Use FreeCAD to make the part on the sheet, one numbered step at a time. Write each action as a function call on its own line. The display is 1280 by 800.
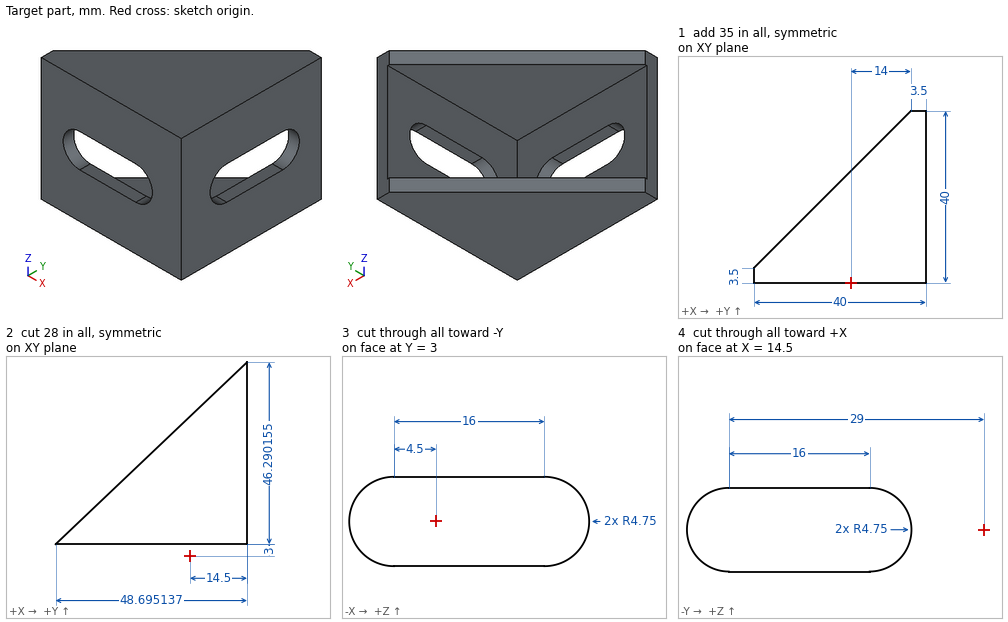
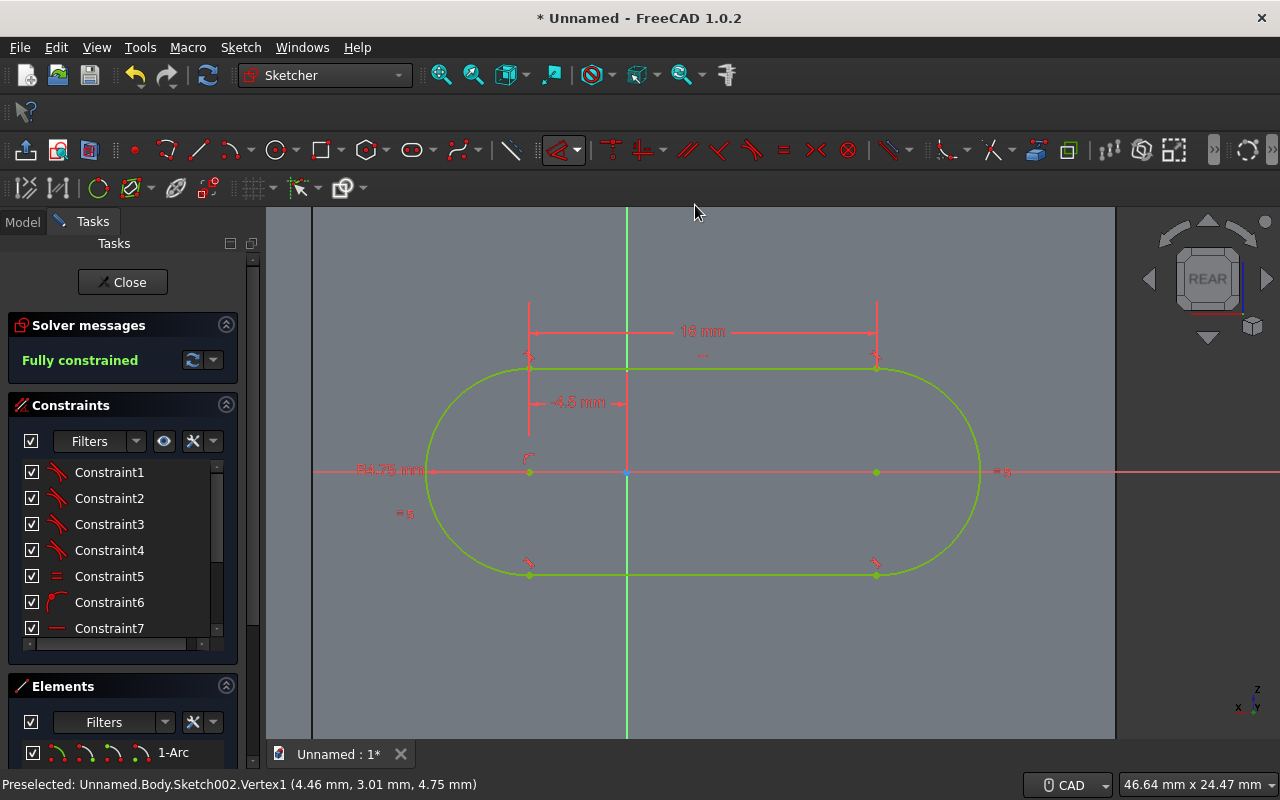
click(123, 282)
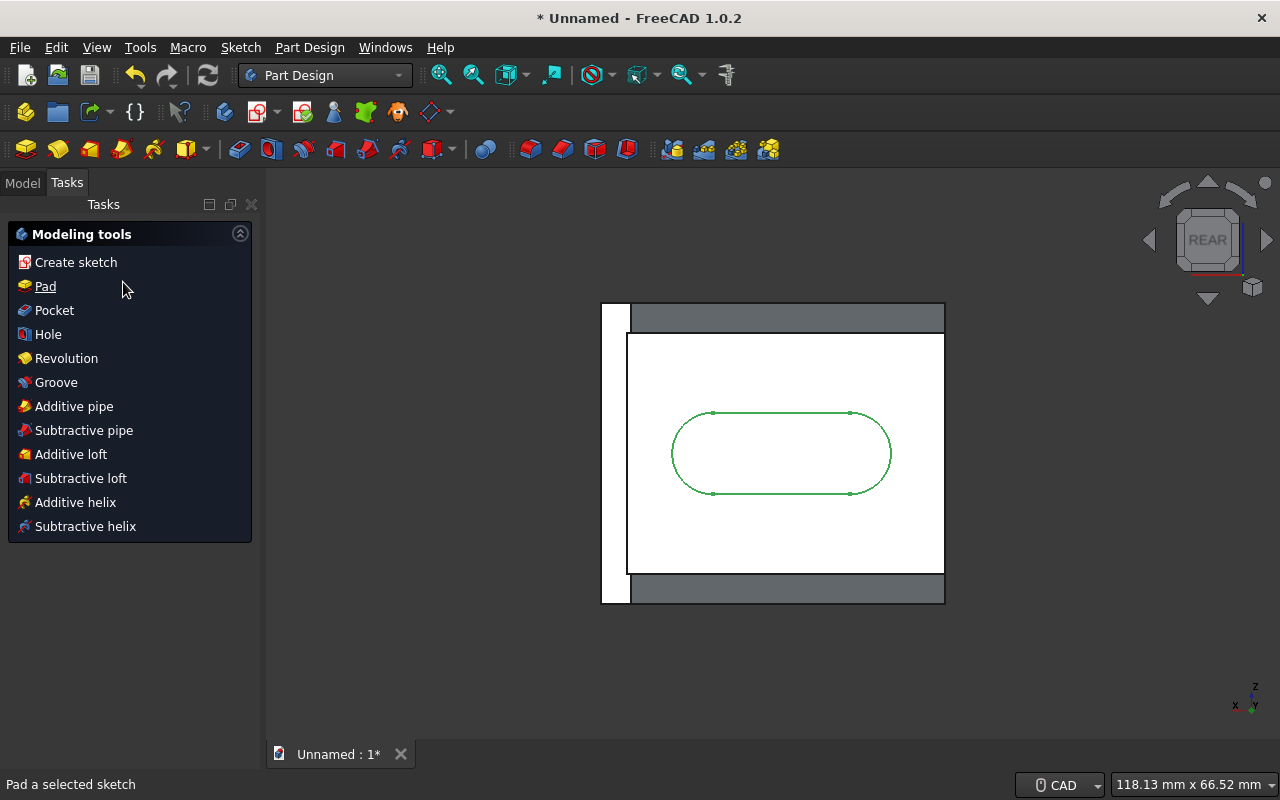
click(240, 150)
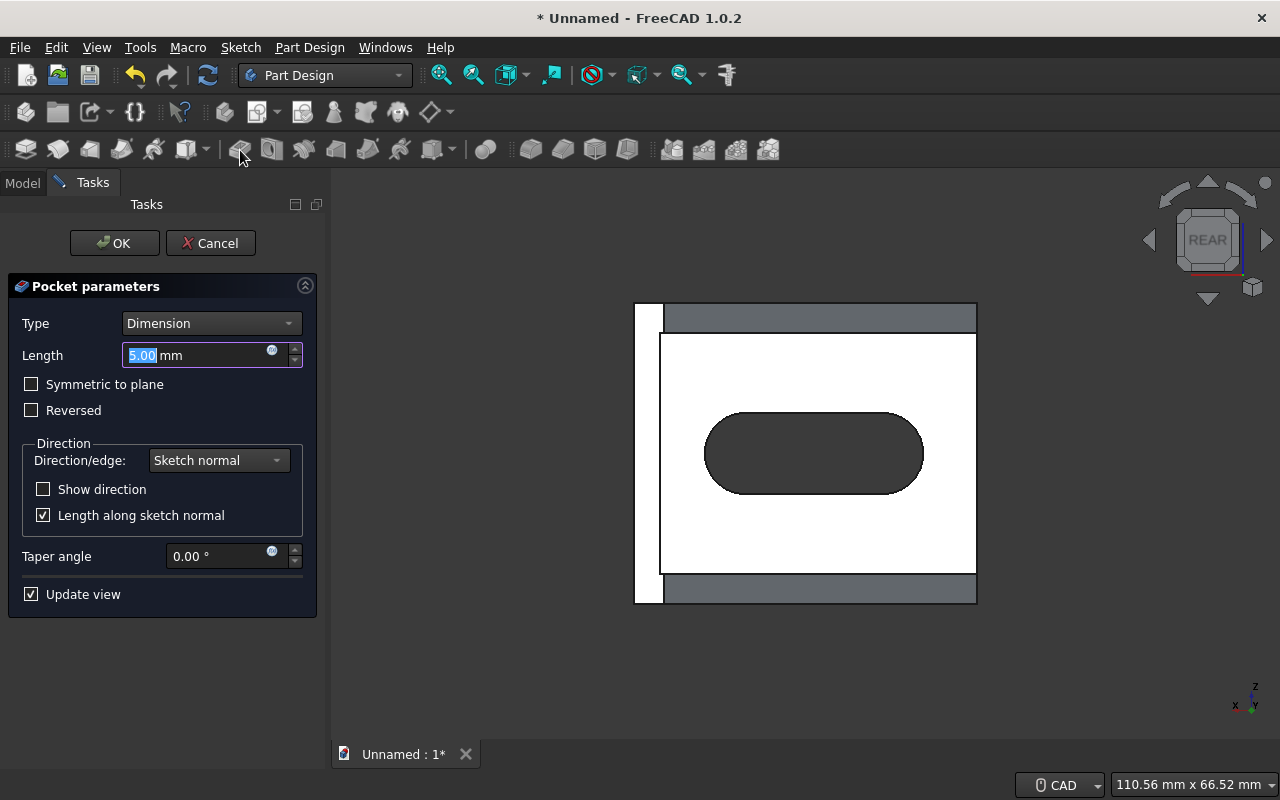
click(212, 324)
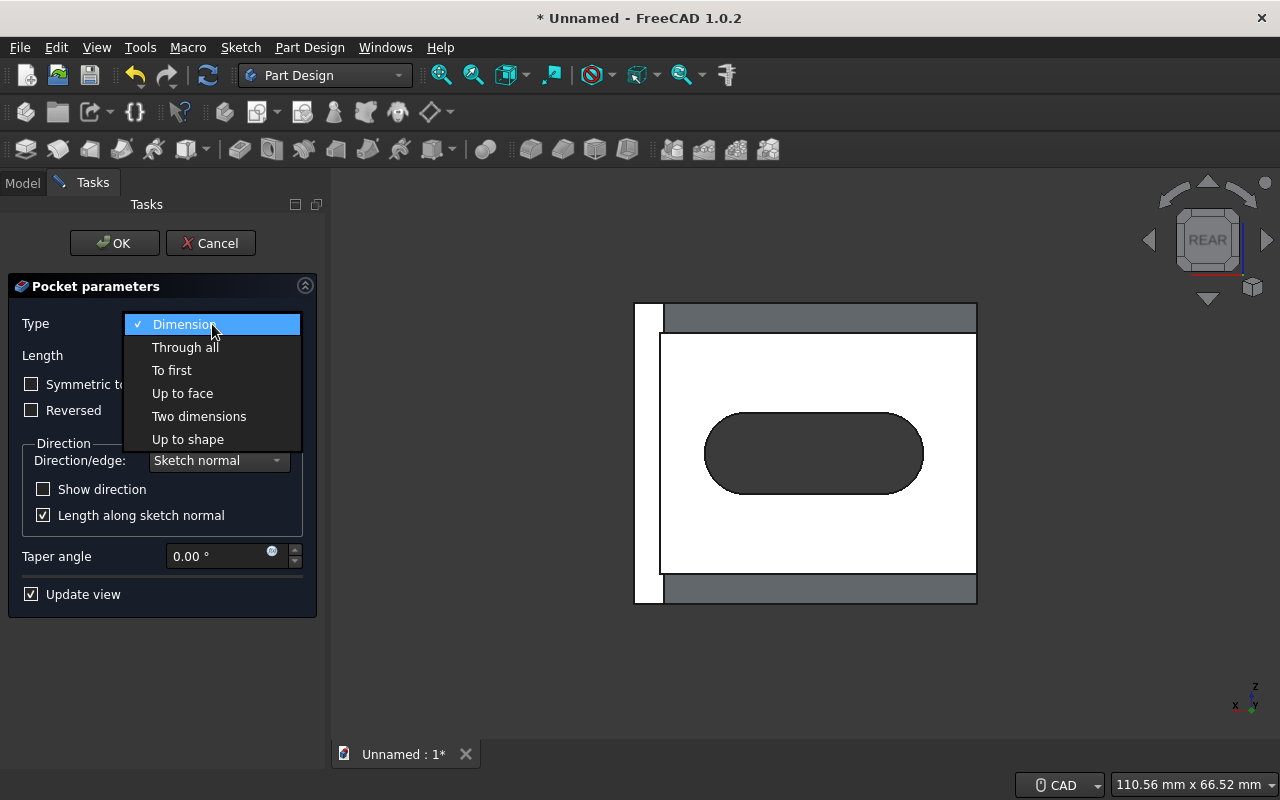
click(212, 348)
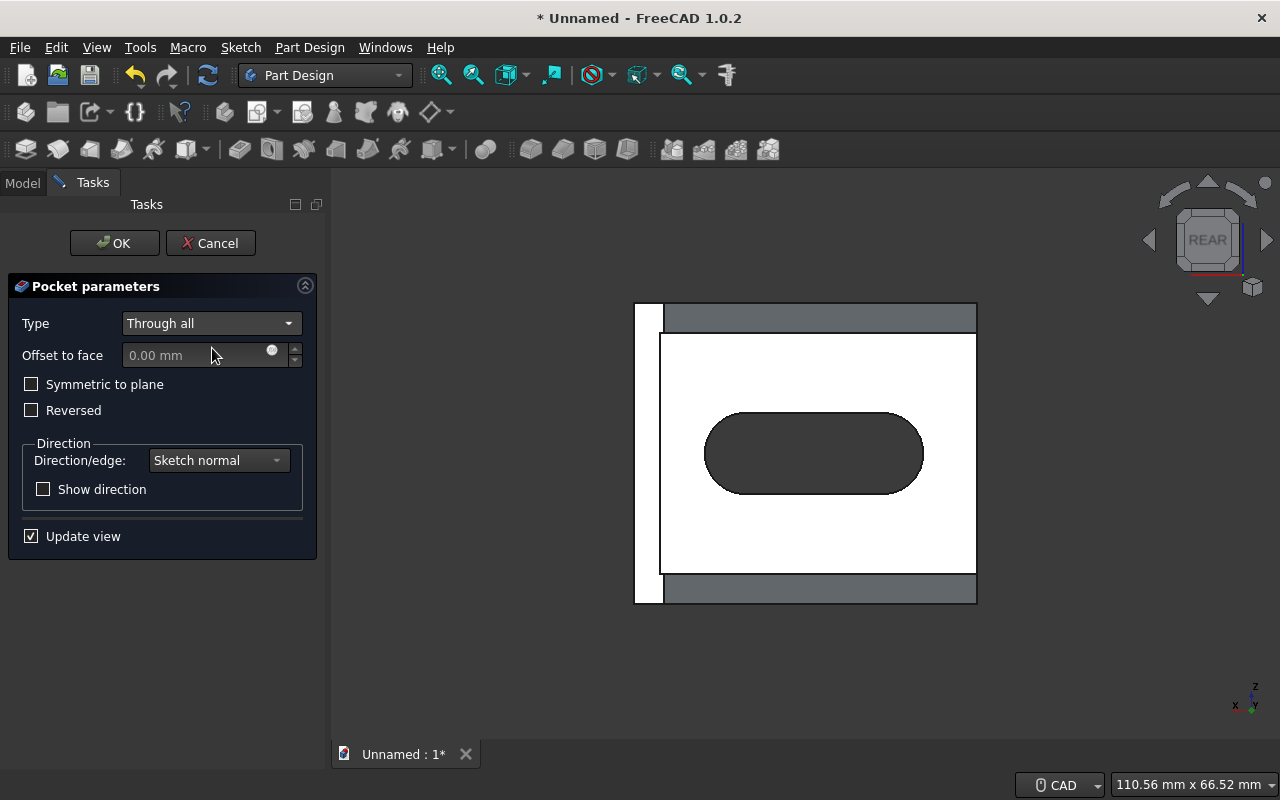
click(115, 243)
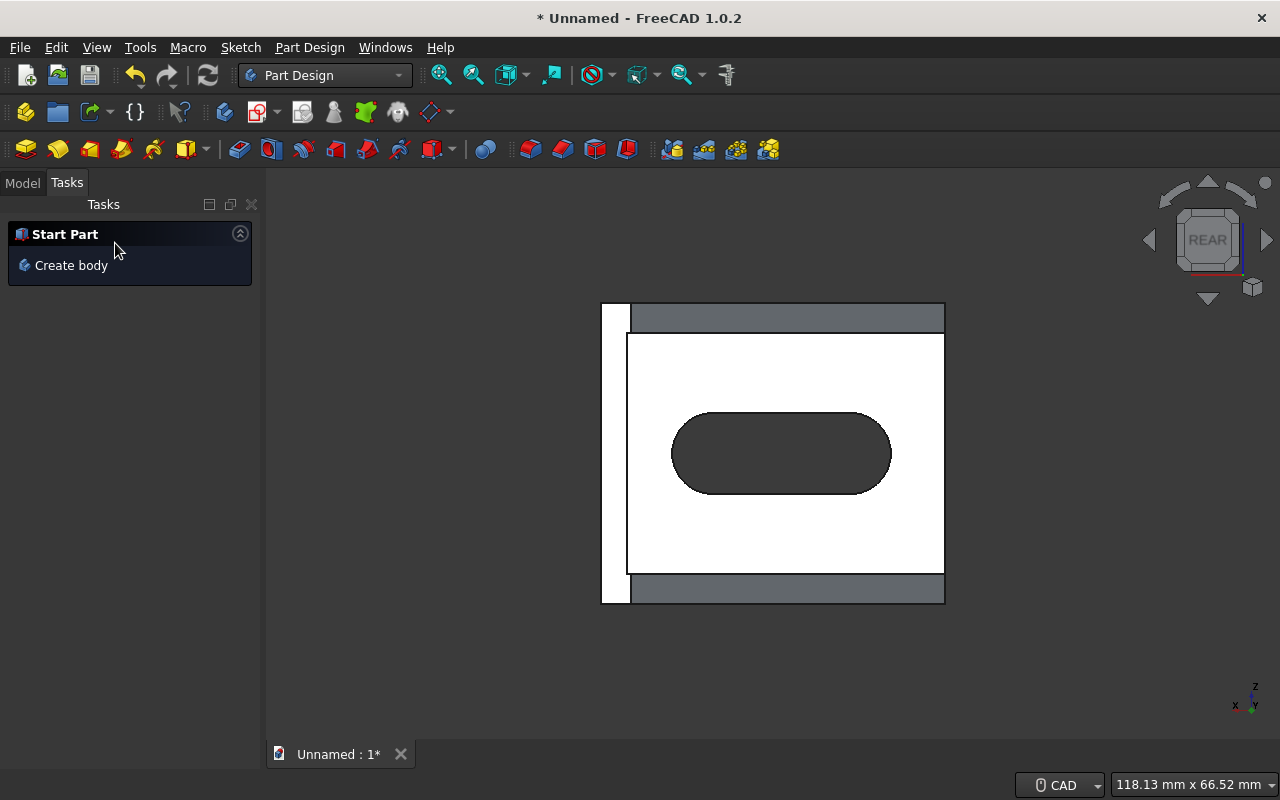
key(6)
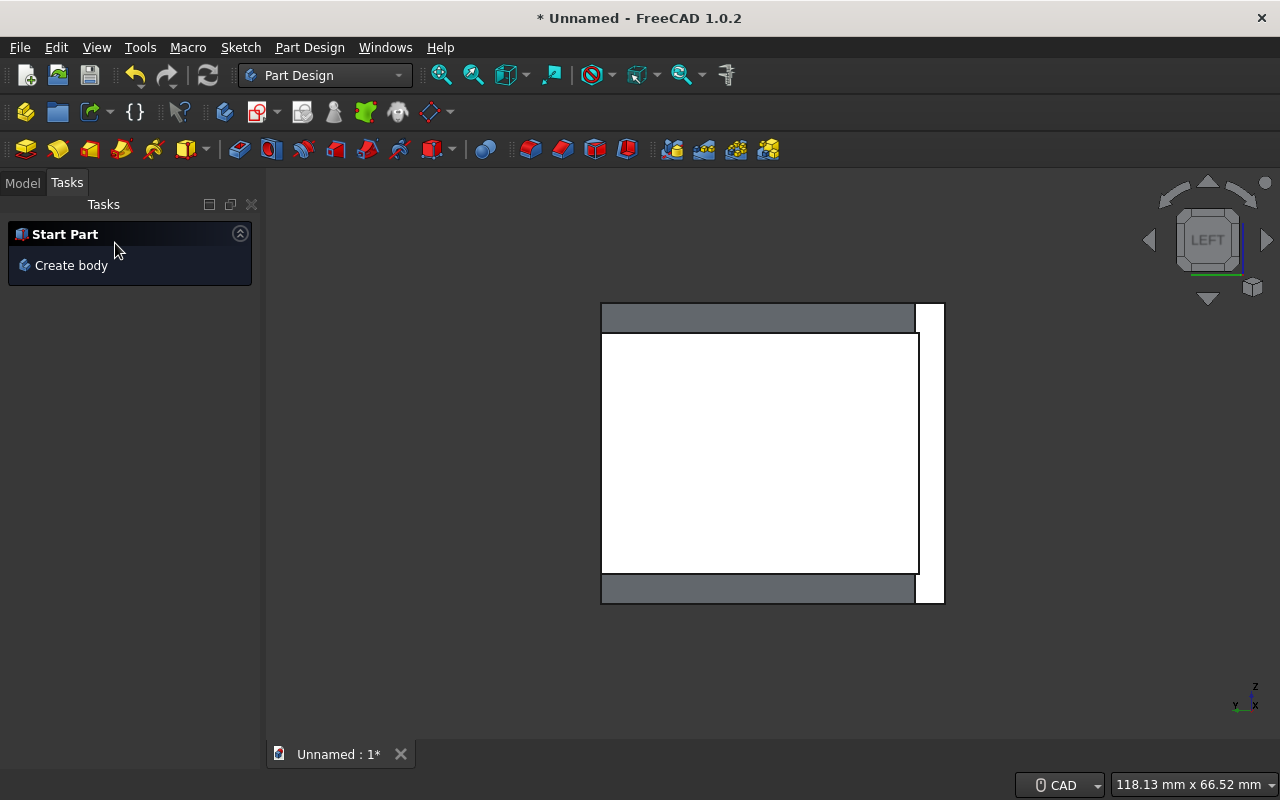
click(760, 453)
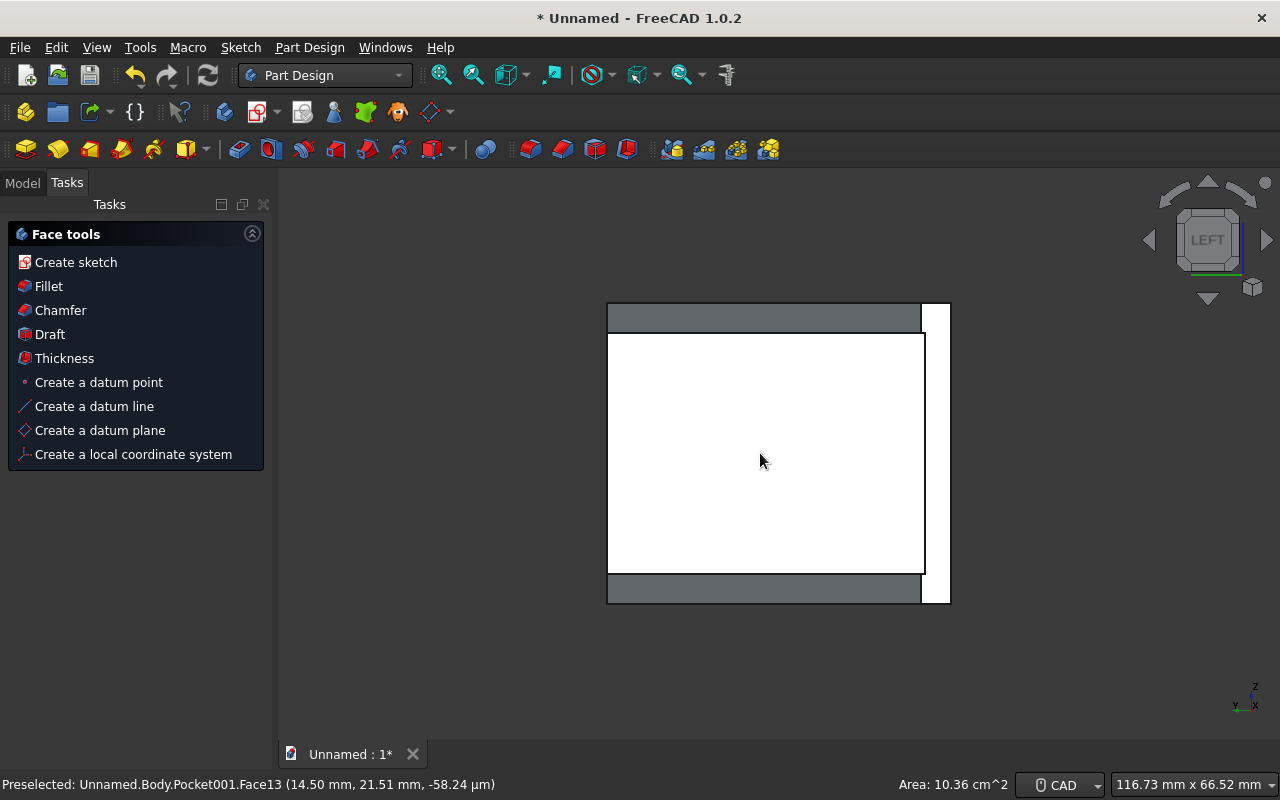
click(258, 112)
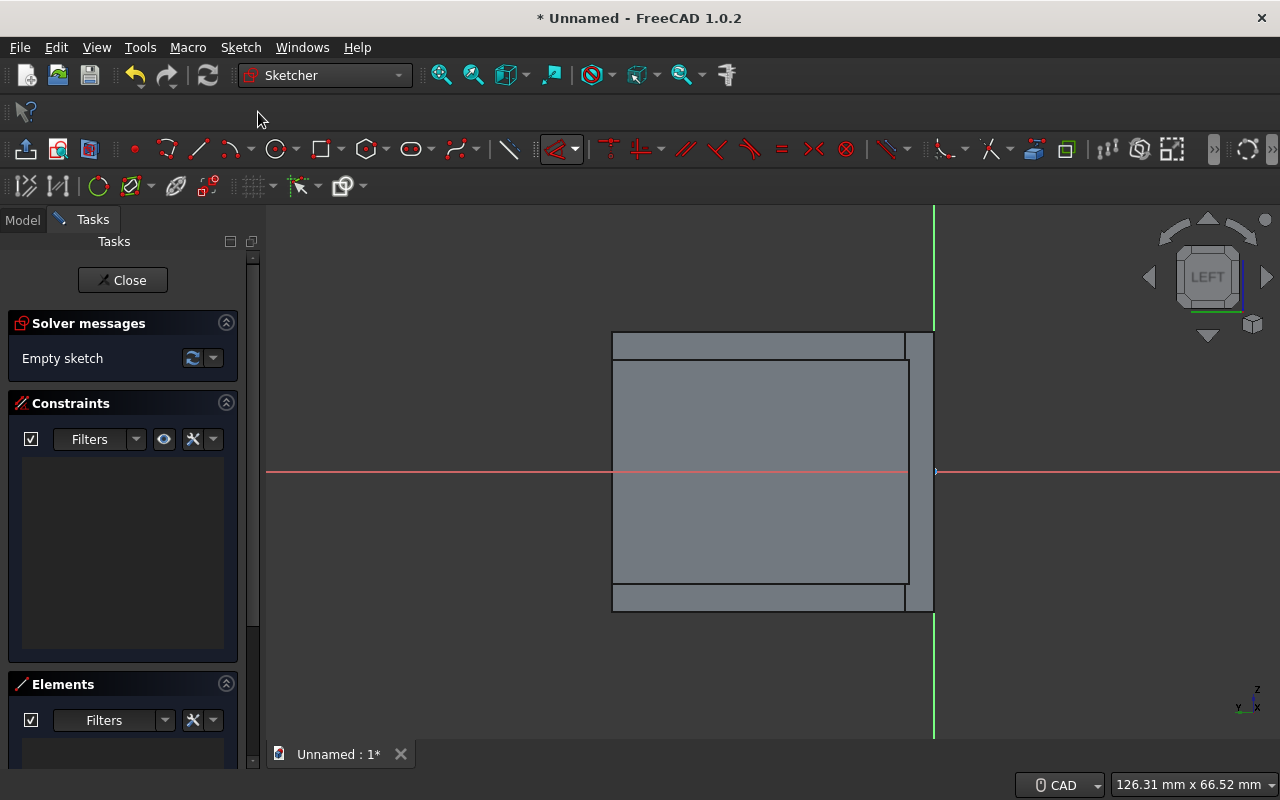
scroll(874, 472, up, 4)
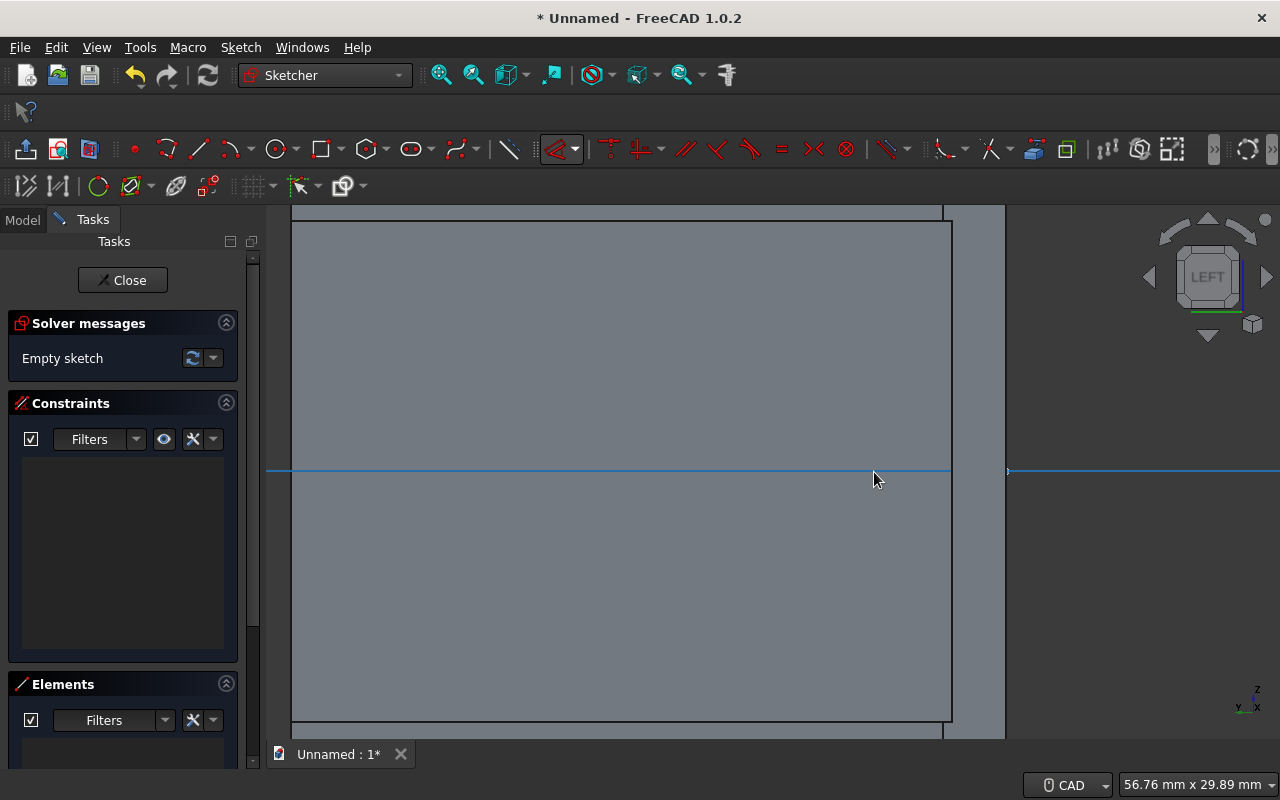
key(g)
key(s)